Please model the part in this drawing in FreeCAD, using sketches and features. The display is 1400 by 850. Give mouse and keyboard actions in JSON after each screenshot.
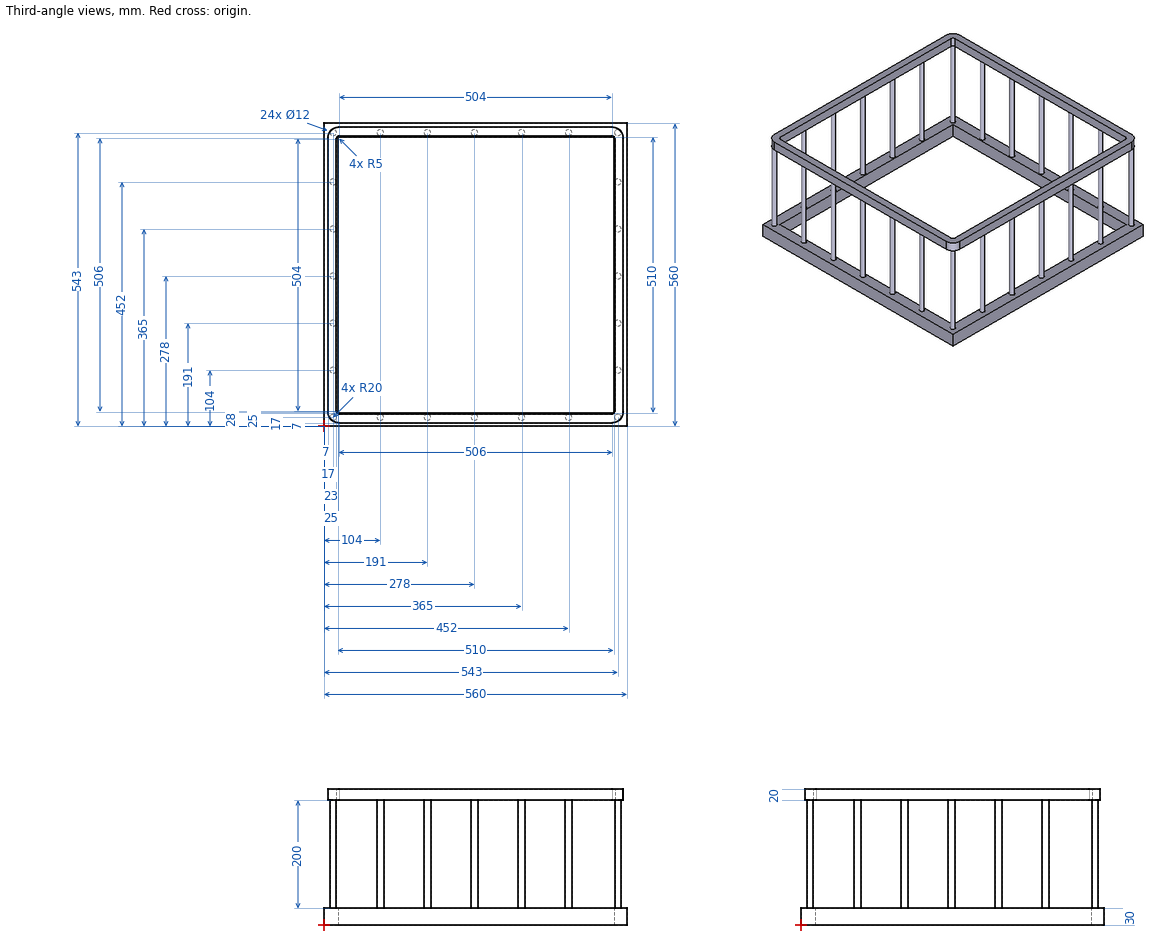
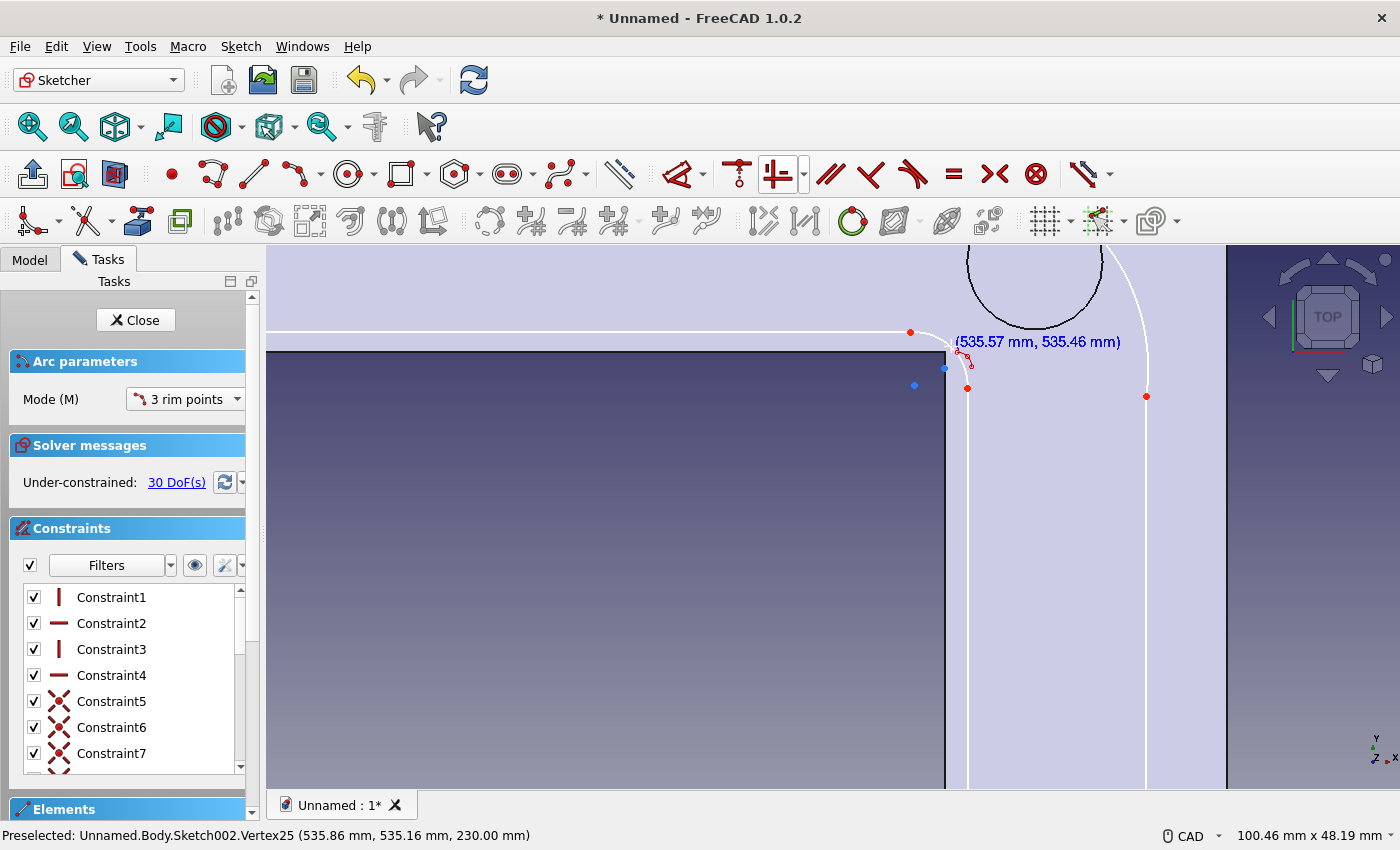
{"action": "scroll", "coordinate": [942, 339], "scroll_direction": "down", "scroll_amount": 14}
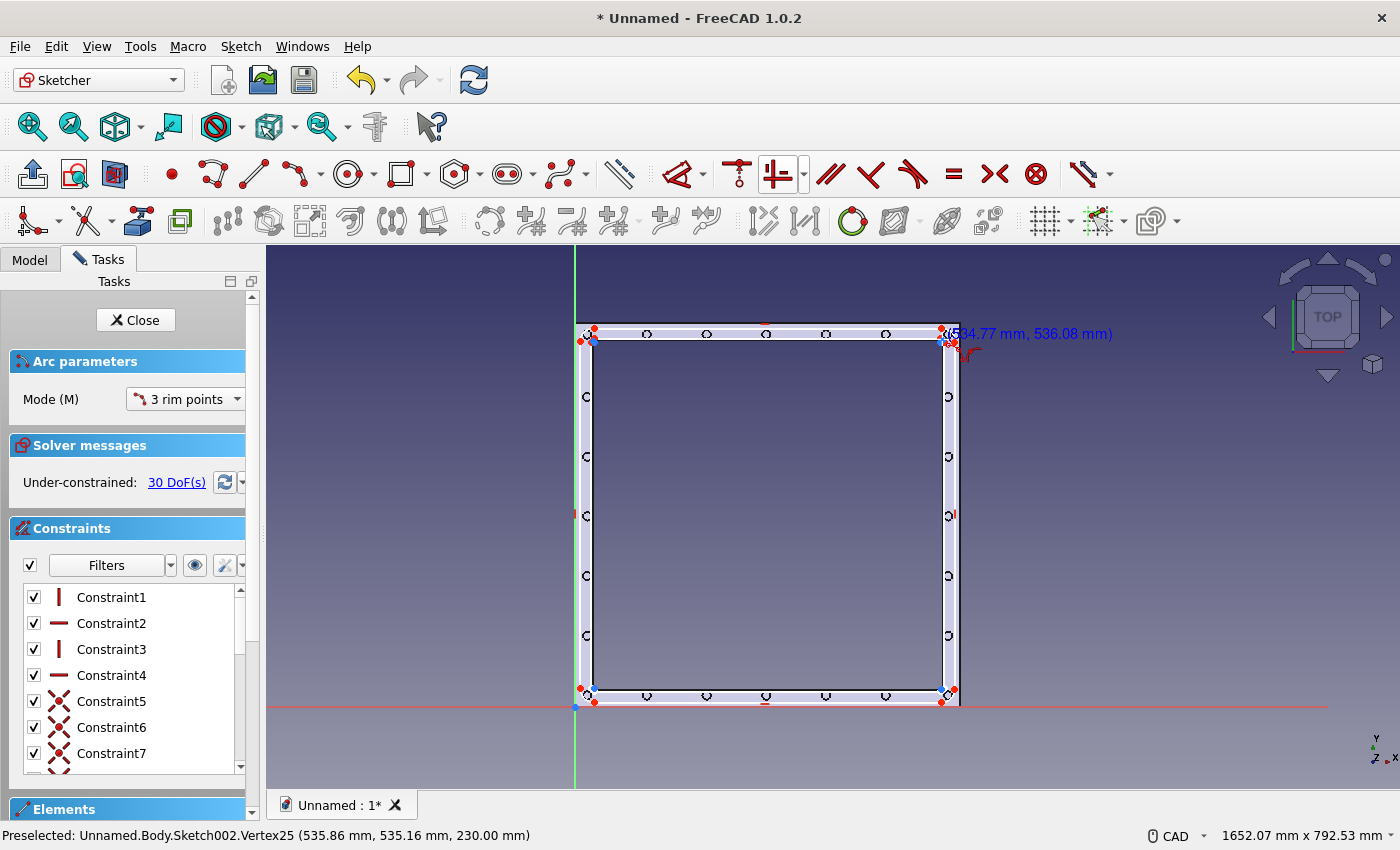
{"action": "scroll", "coordinate": [944, 688], "scroll_direction": "up", "scroll_amount": 9}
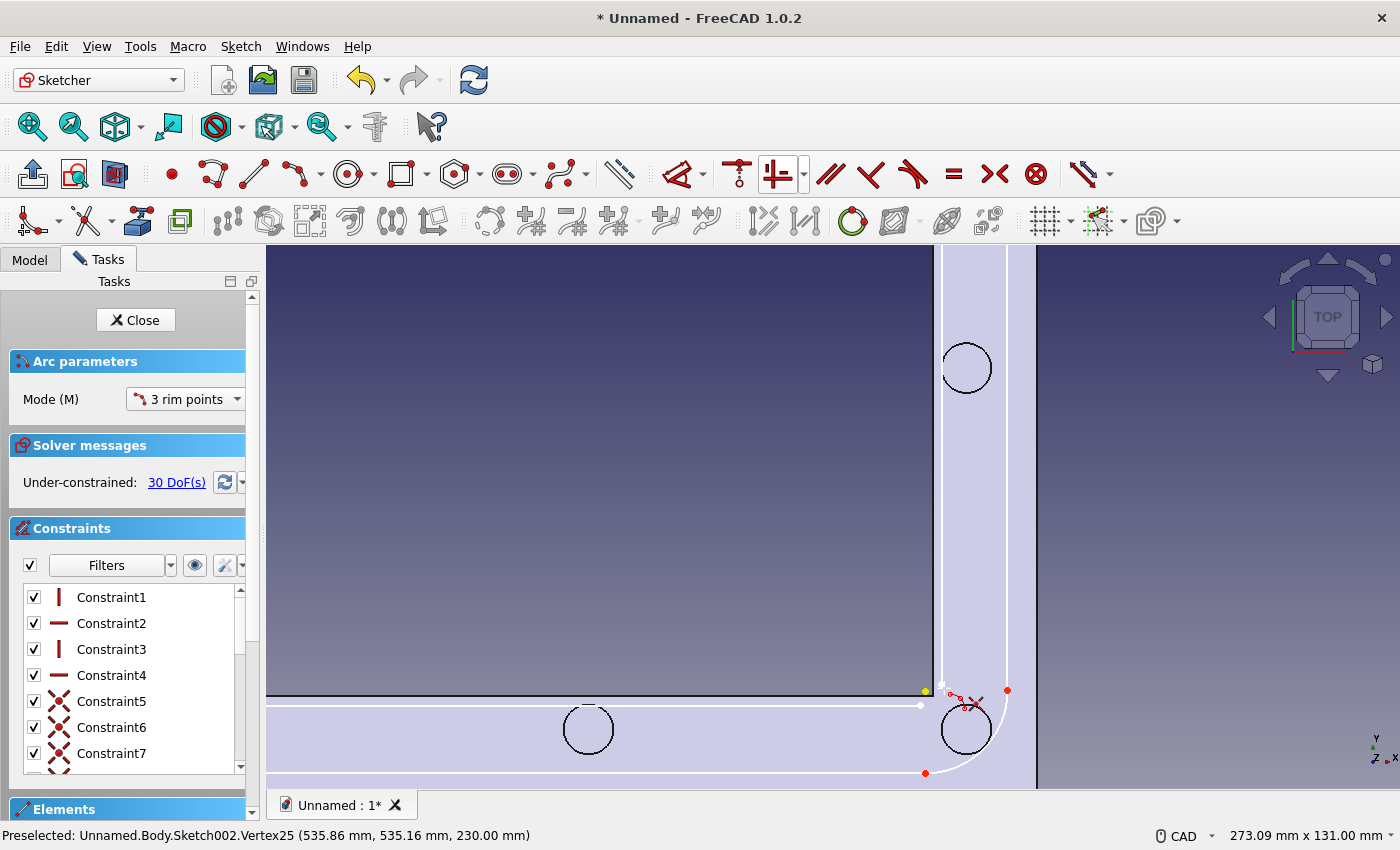
{"action": "left_click", "coordinate": [942, 685]}
{"action": "left_click", "coordinate": [921, 706]}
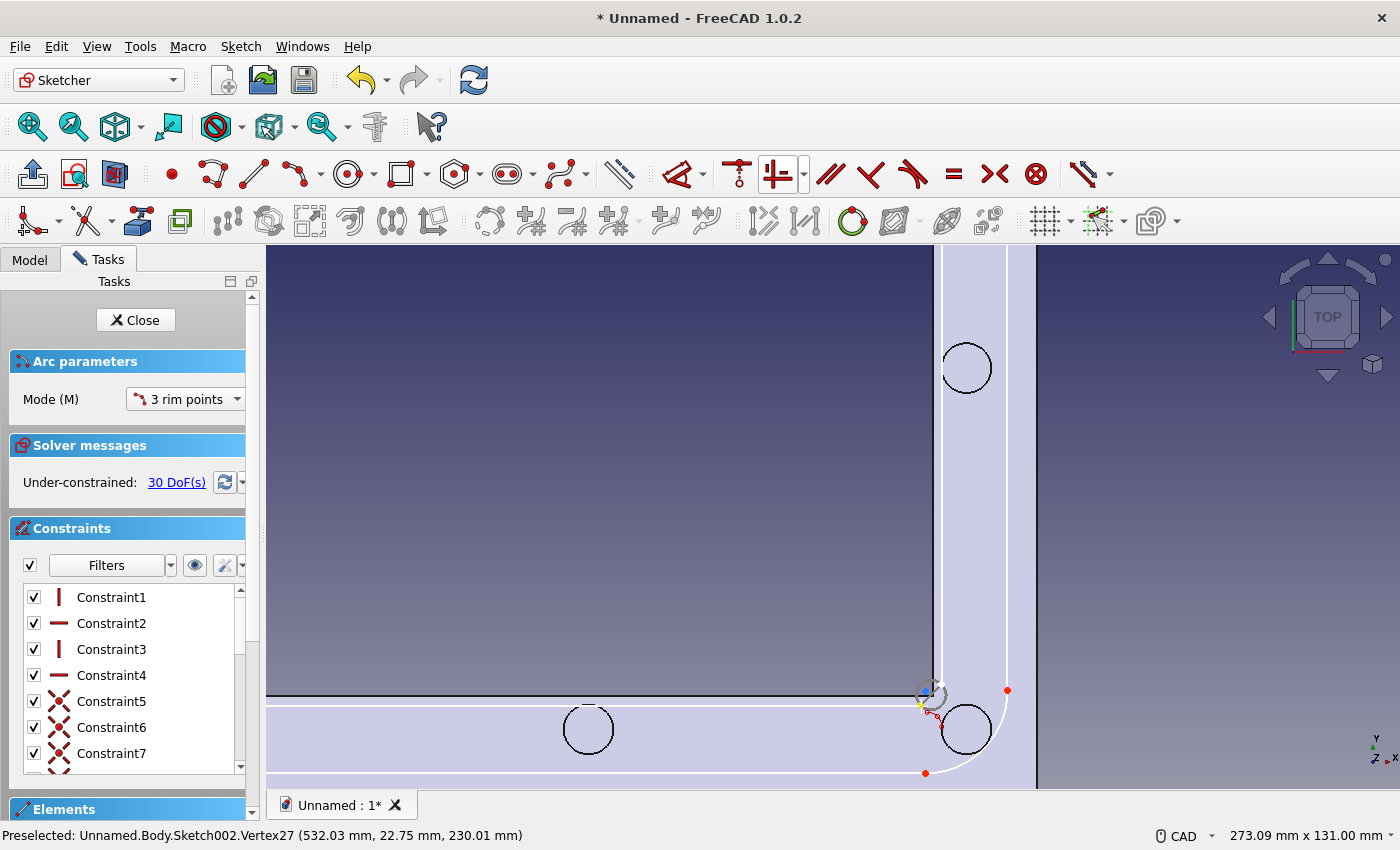
{"action": "scroll", "coordinate": [935, 698], "scroll_direction": "up", "scroll_amount": 5}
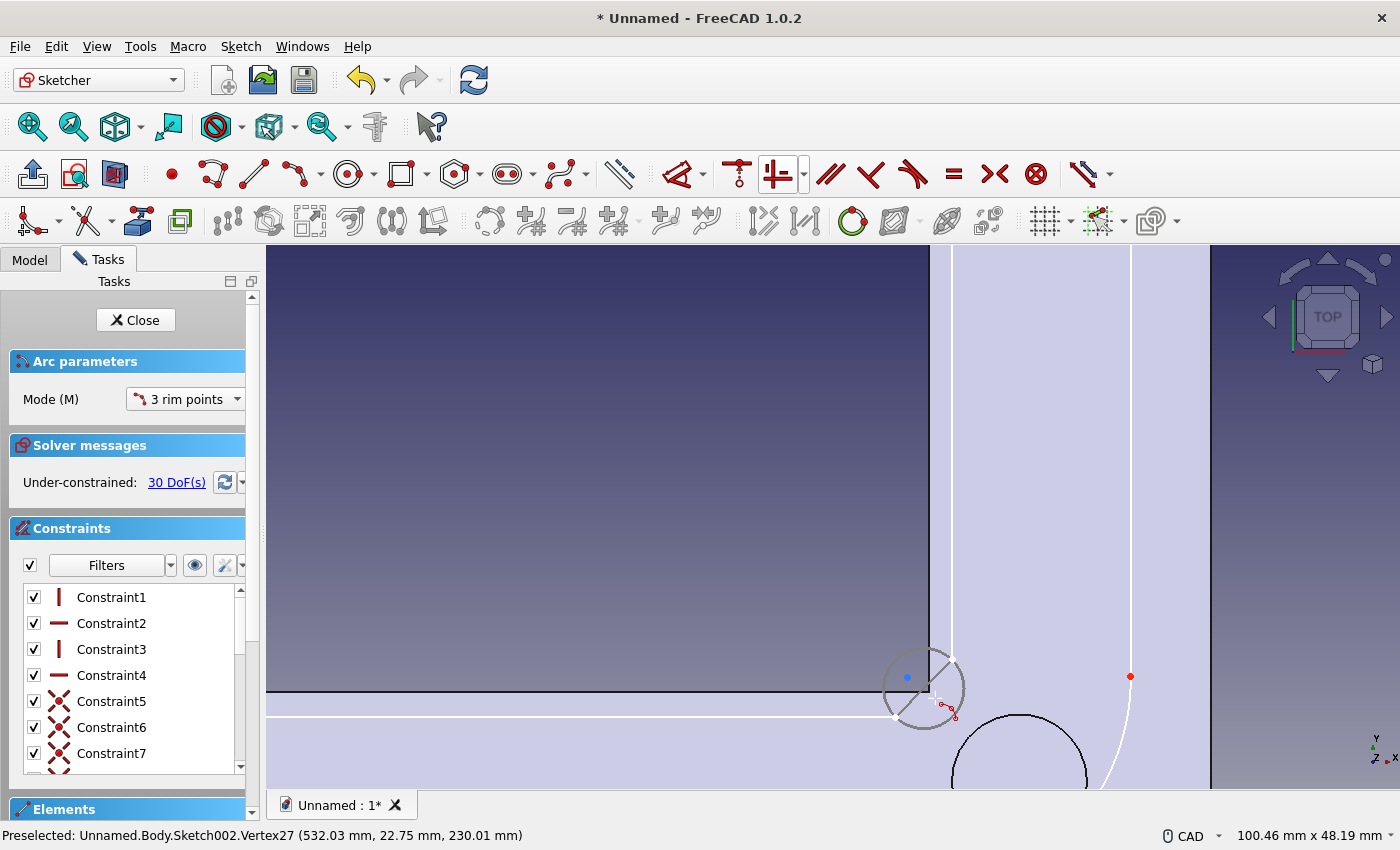
{"action": "left_click", "coordinate": [935, 698]}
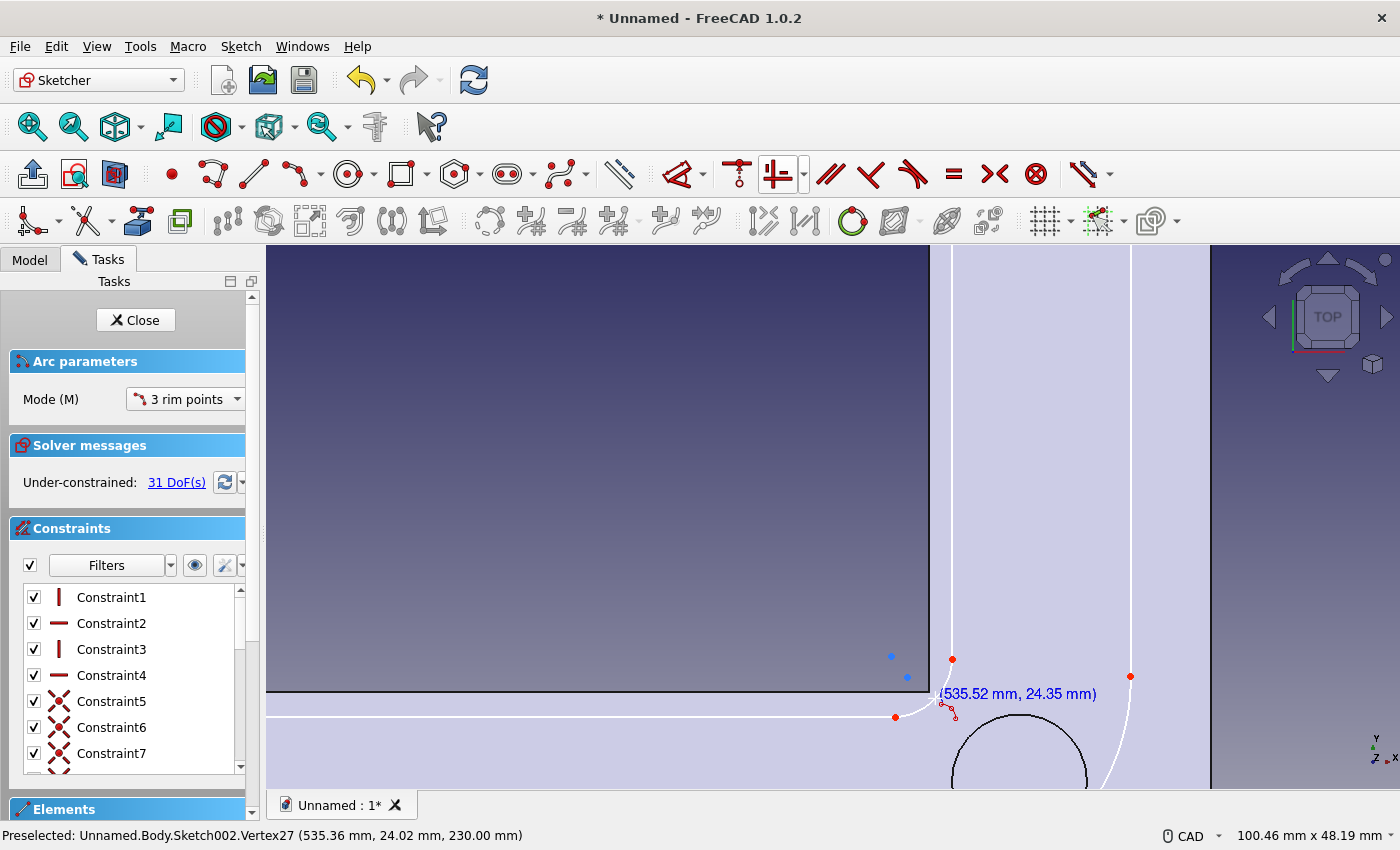
{"action": "scroll", "coordinate": [943, 689], "scroll_direction": "down", "scroll_amount": 14}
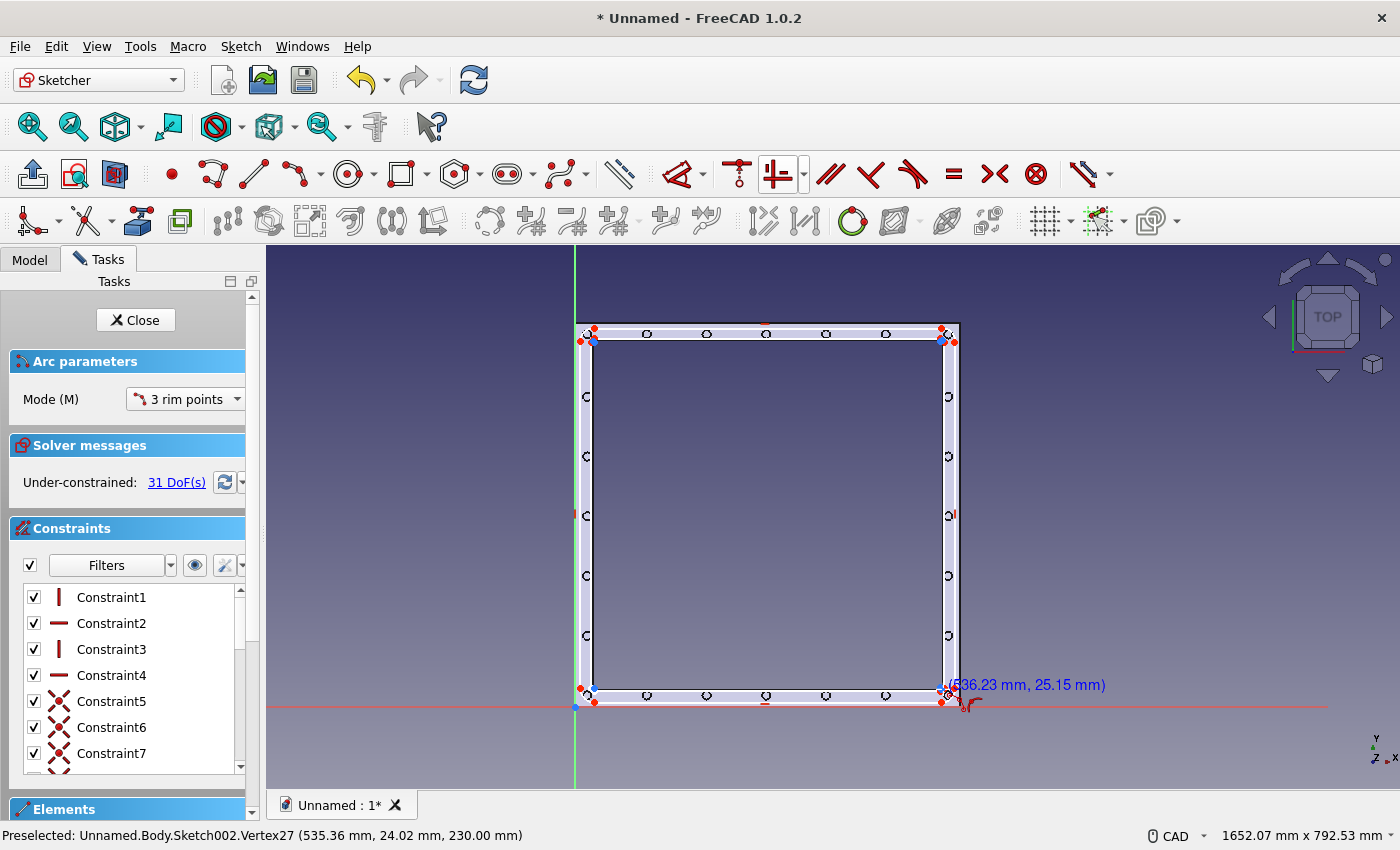
{"action": "scroll", "coordinate": [595, 691], "scroll_direction": "up", "scroll_amount": 9}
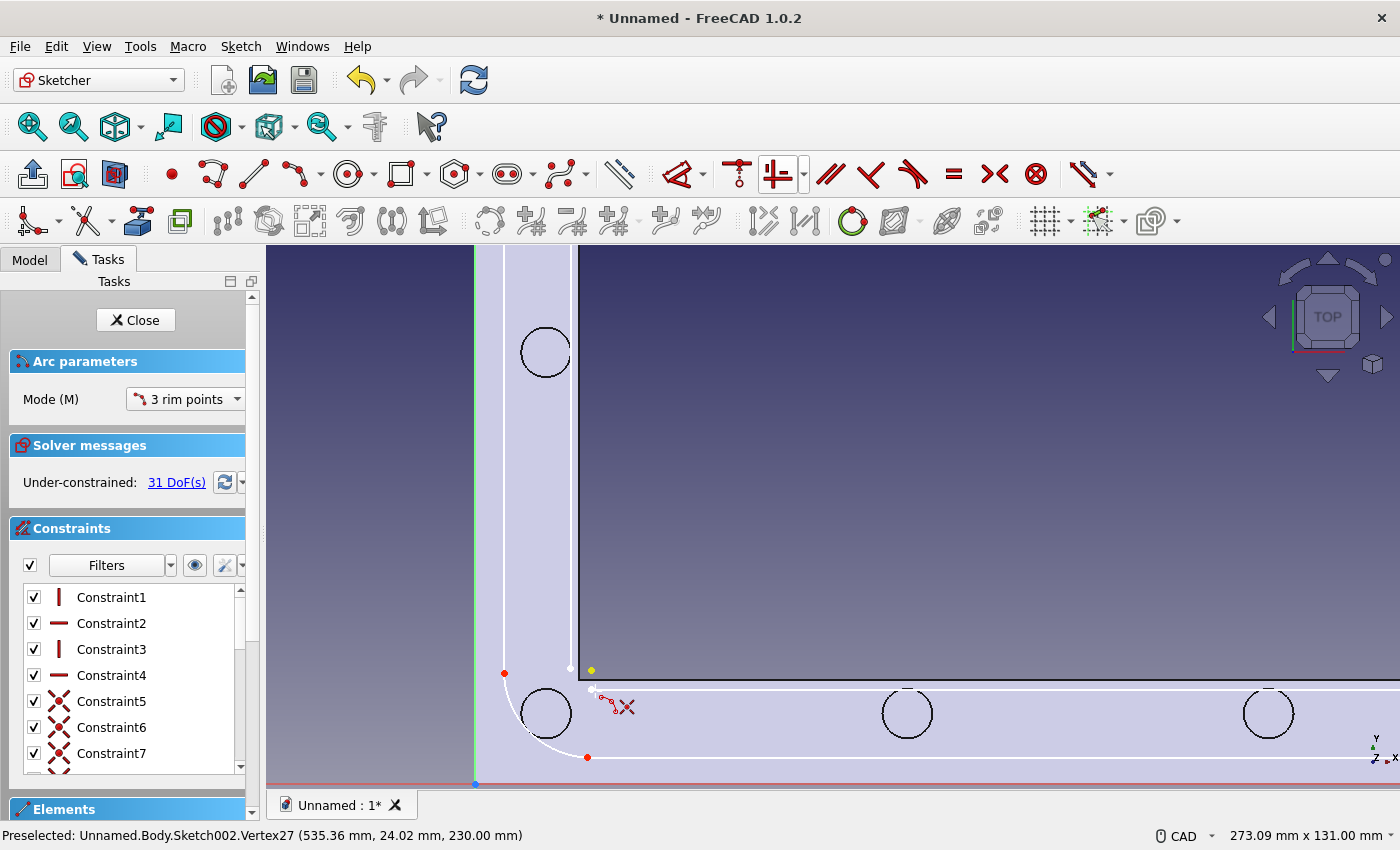
{"action": "left_click", "coordinate": [592, 690]}
{"action": "left_click", "coordinate": [571, 669]}